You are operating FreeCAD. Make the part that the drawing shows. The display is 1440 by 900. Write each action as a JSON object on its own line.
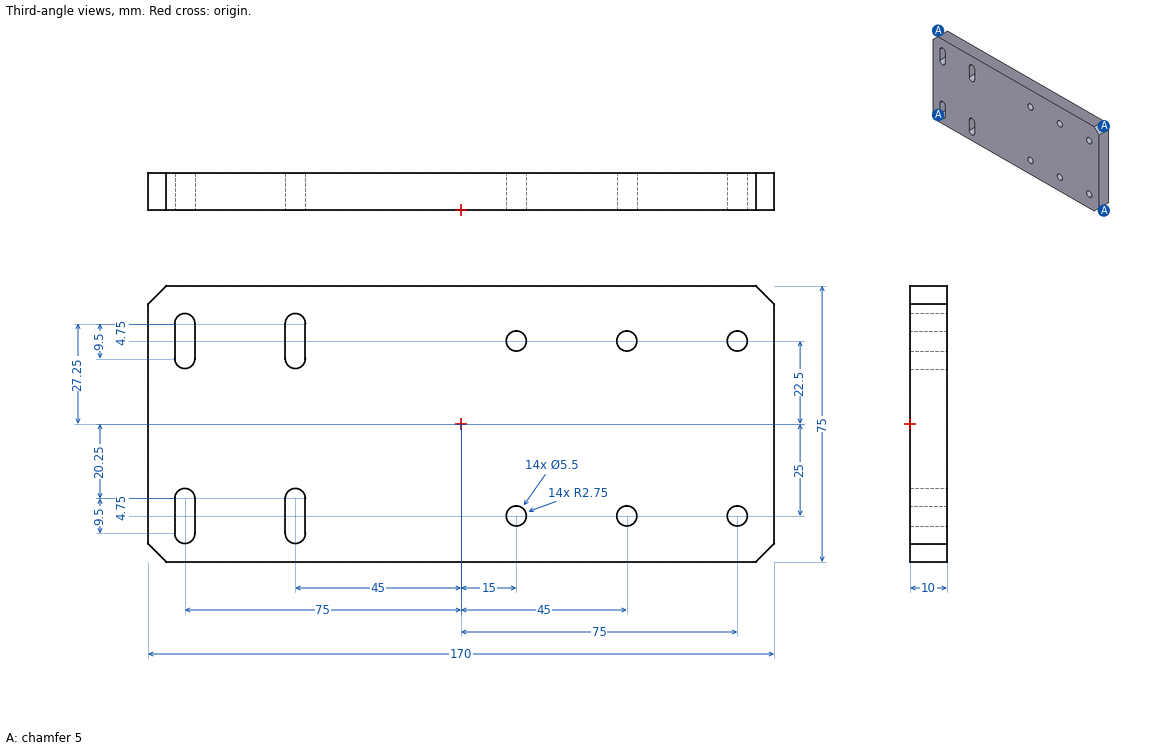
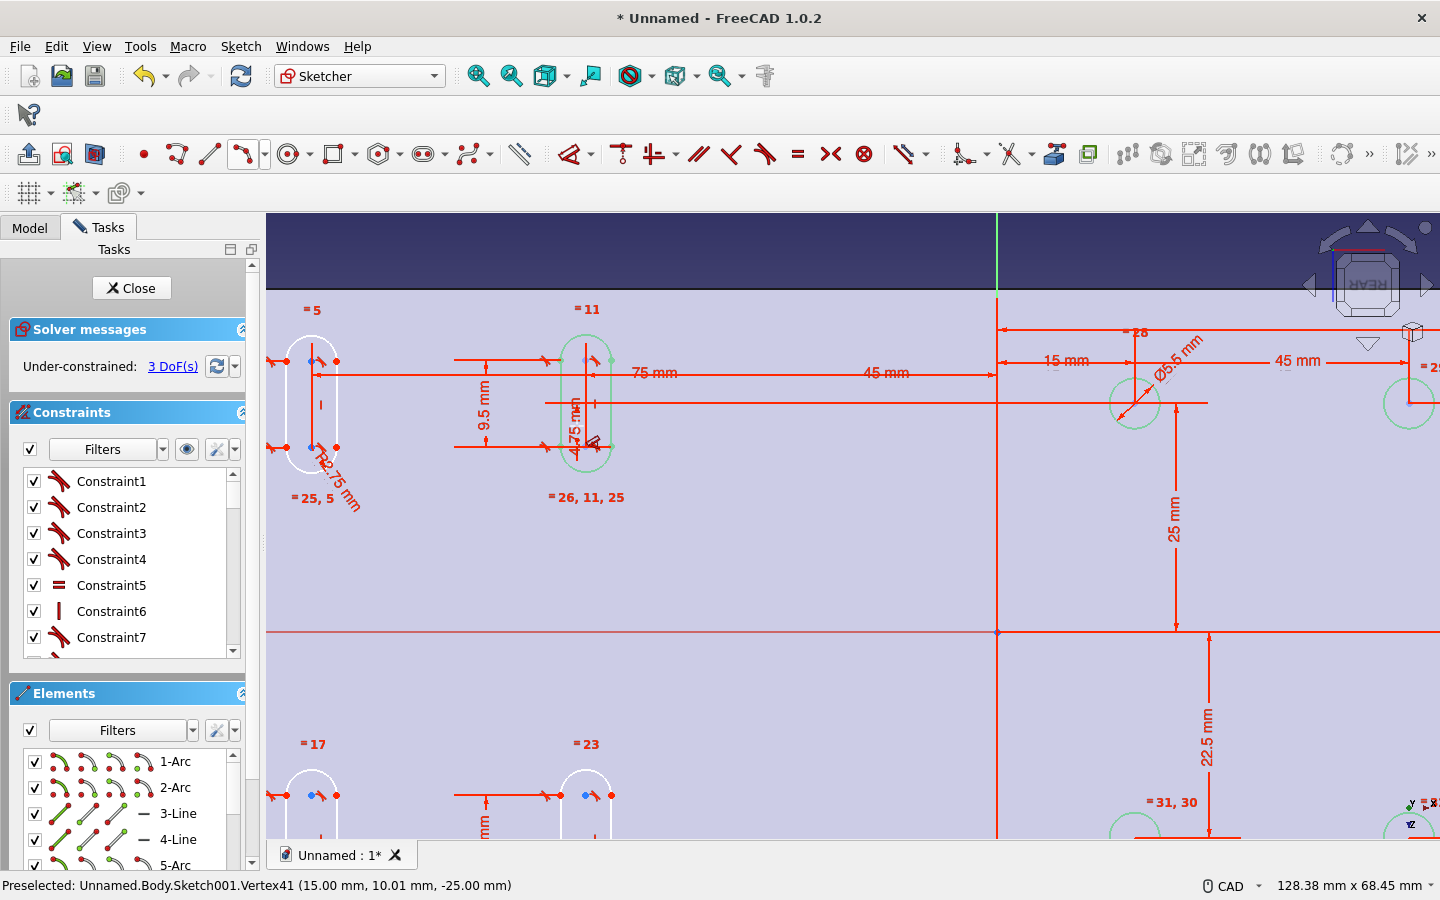
{"action": "scroll", "coordinate": [611, 449], "scroll_direction": "down", "scroll_amount": 4}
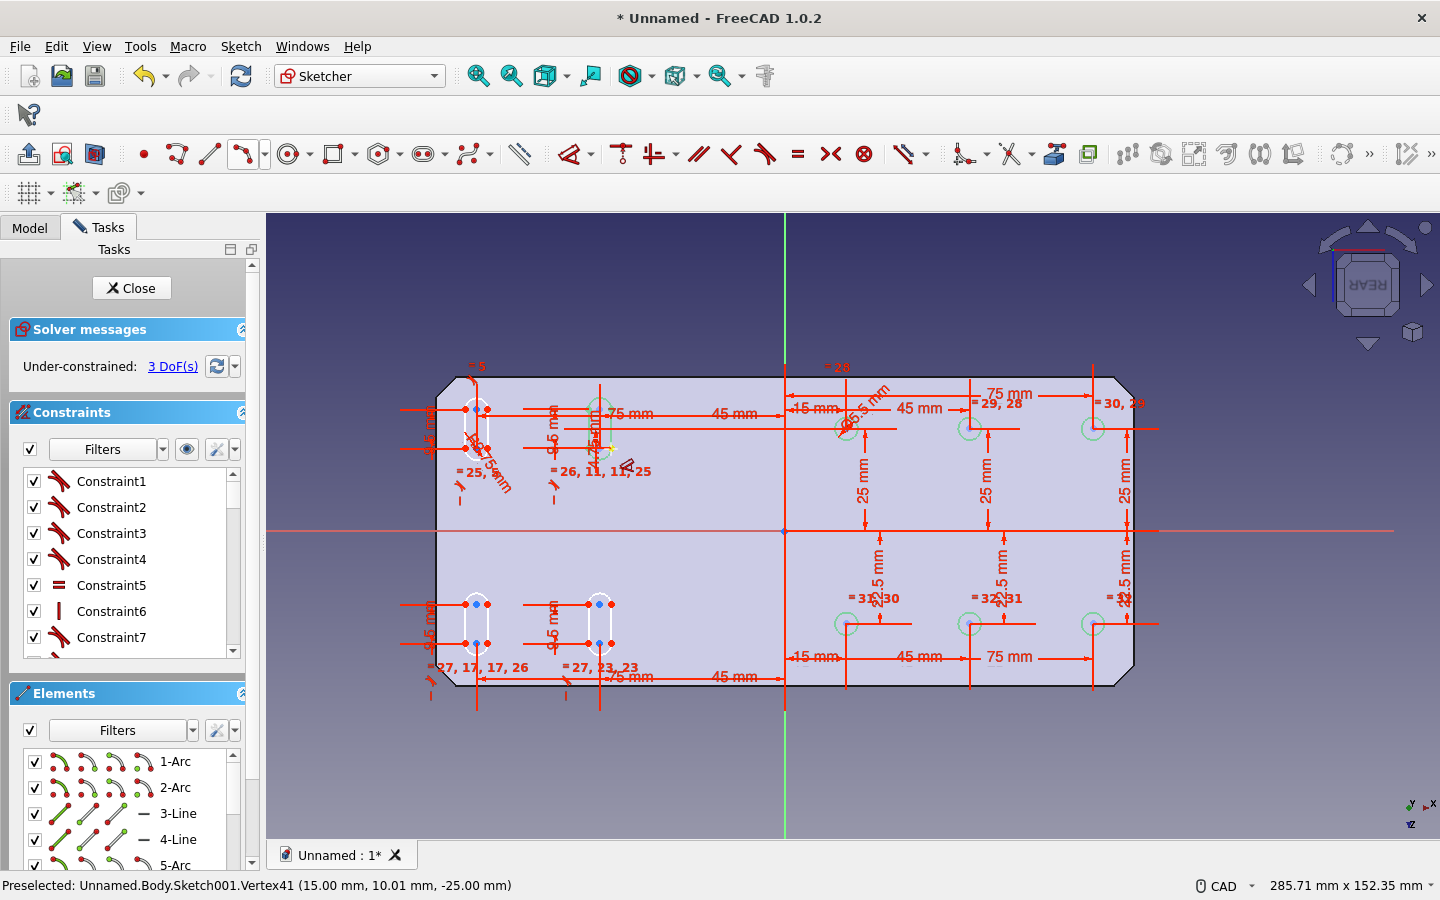
{"action": "scroll", "coordinate": [611, 644], "scroll_direction": "up", "scroll_amount": 4}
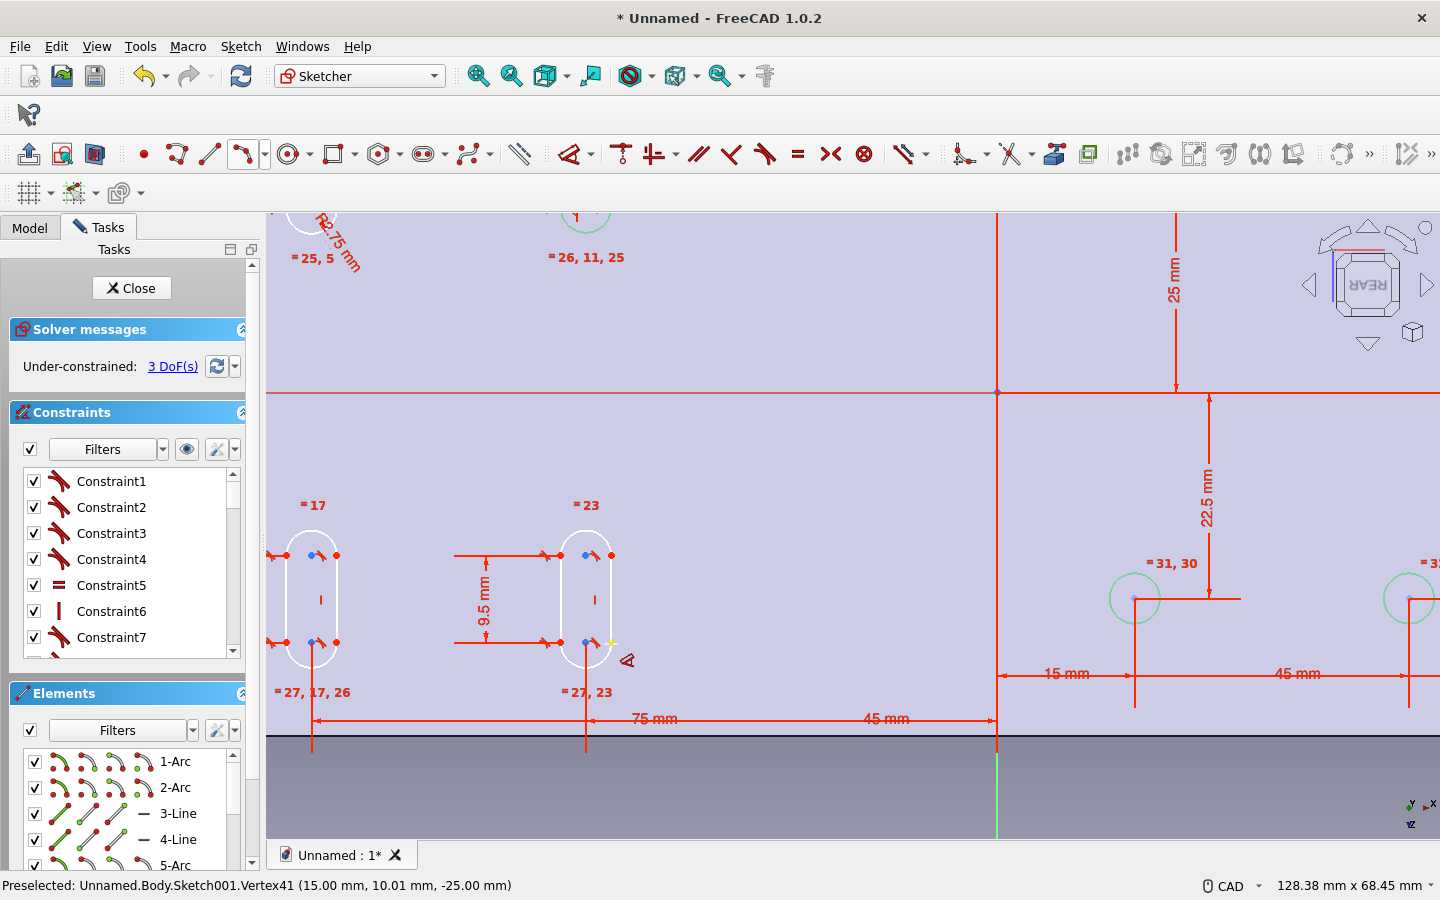
{"action": "left_click", "coordinate": [611, 643]}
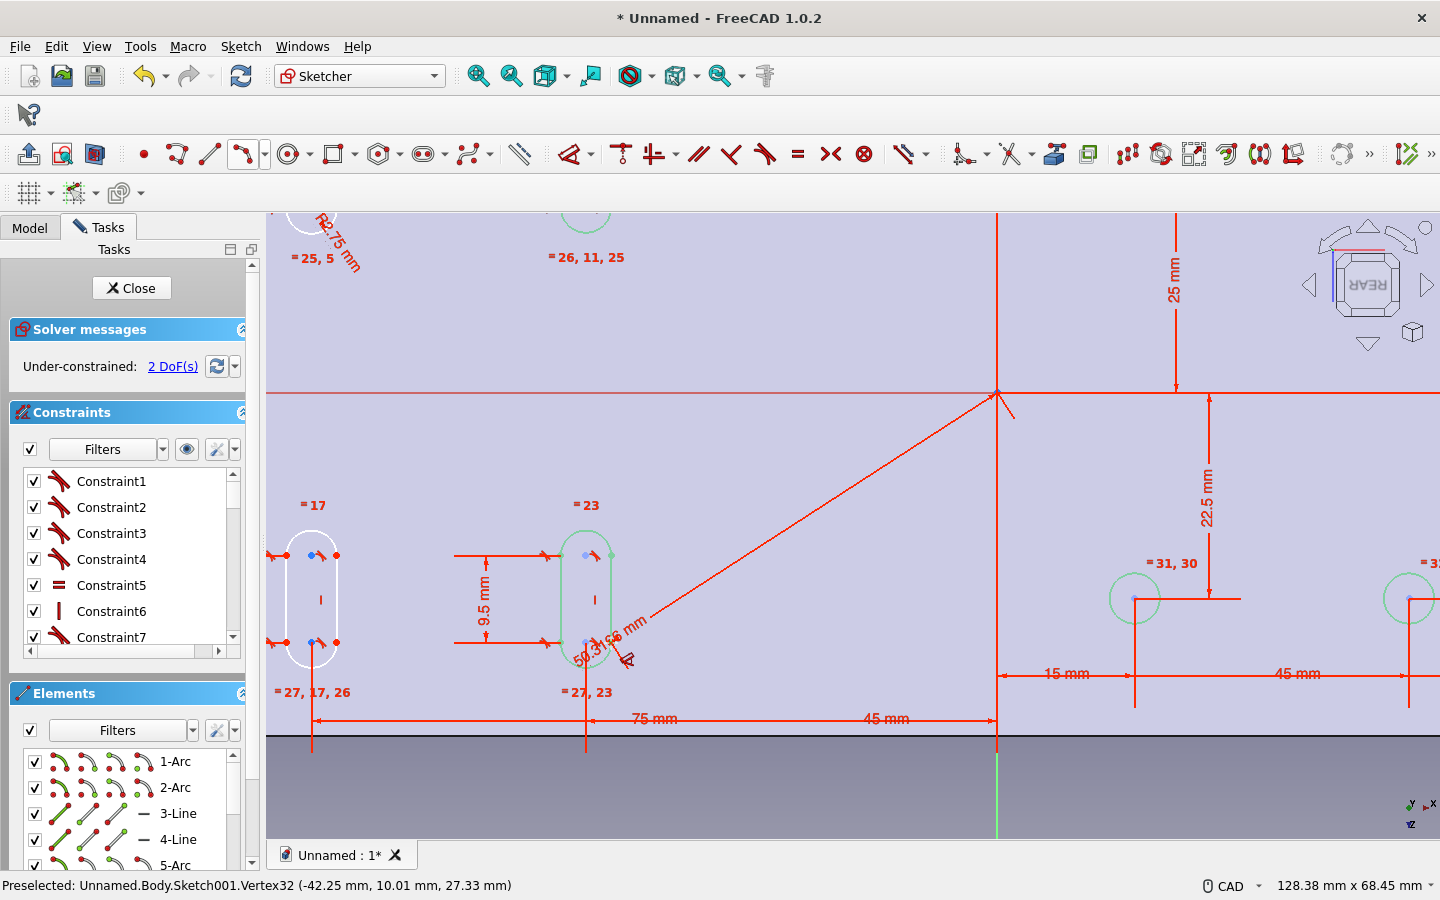
{"action": "left_click", "coordinate": [1135, 598]}
{"action": "left_click", "coordinate": [577, 621]}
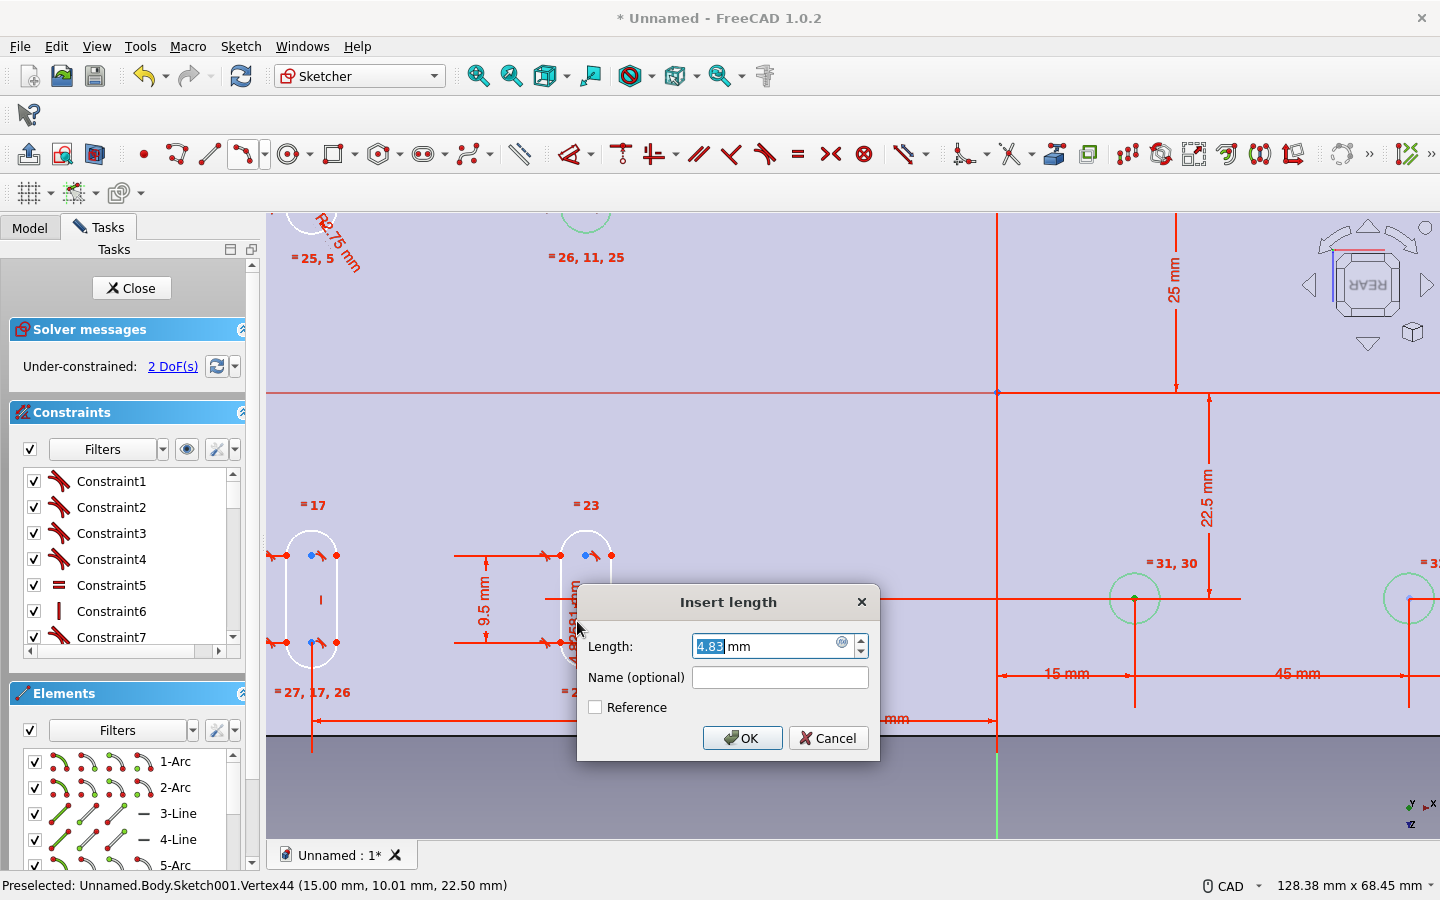
{"action": "type", "text": "4.75"}
{"action": "key", "text": "Return"}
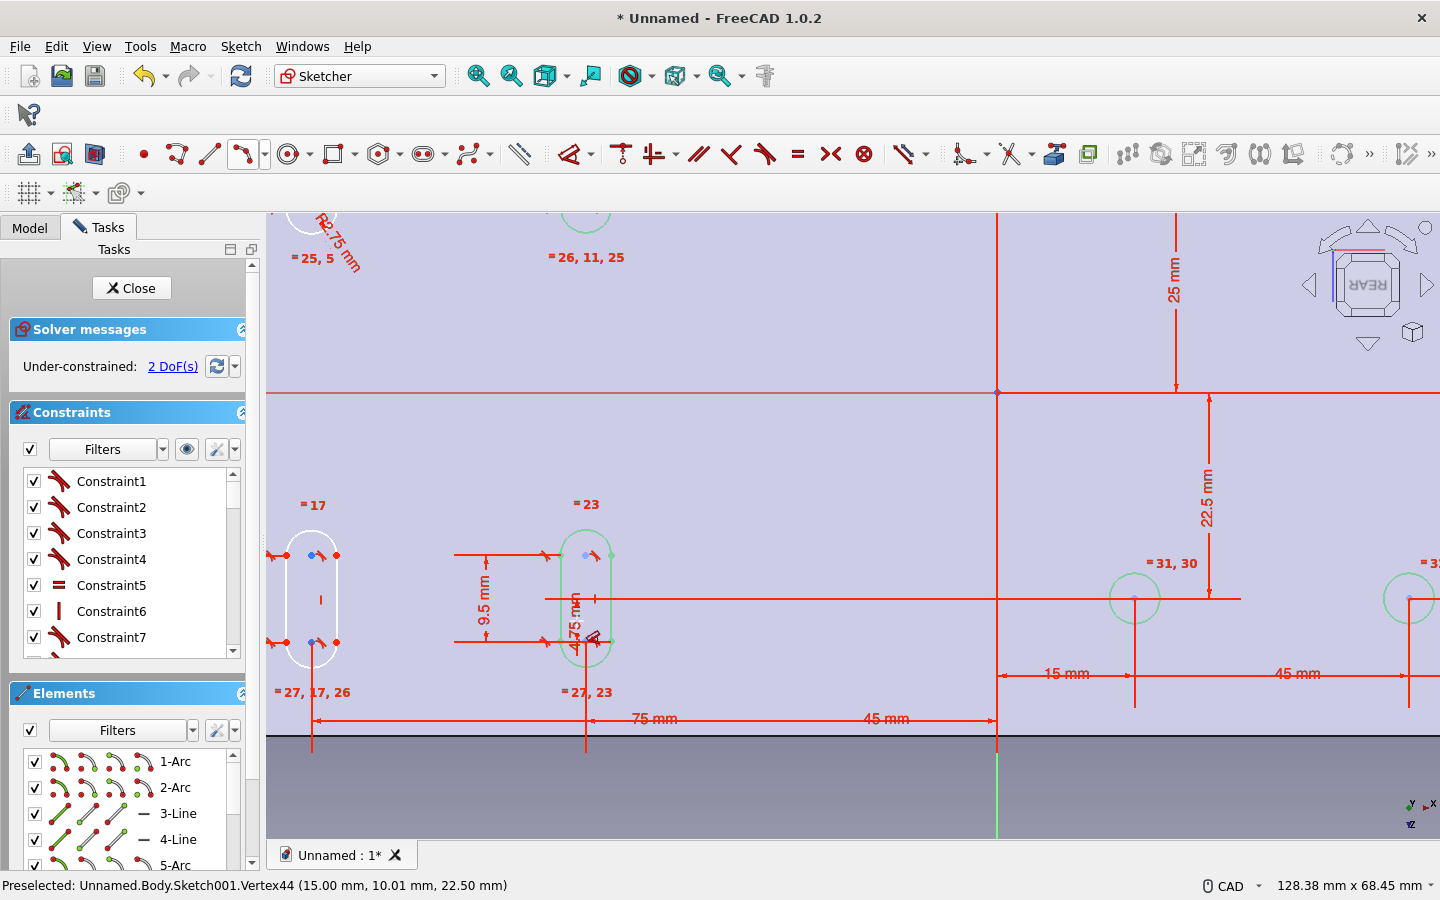
{"action": "scroll", "coordinate": [611, 644], "scroll_direction": "down", "scroll_amount": 4}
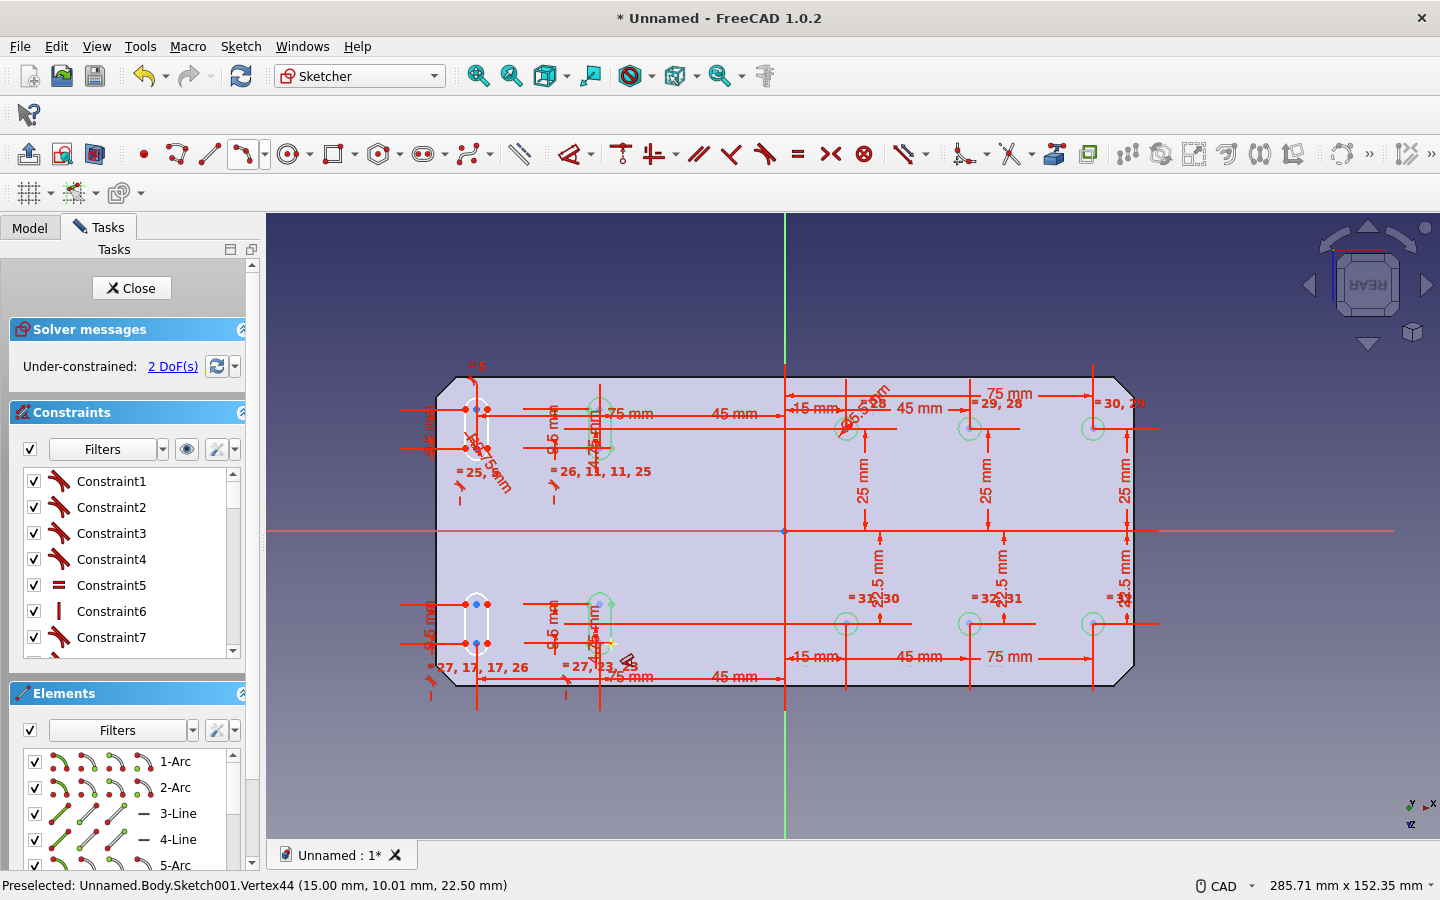
{"action": "left_click", "coordinate": [465, 449]}
{"action": "left_click", "coordinate": [431, 490]}